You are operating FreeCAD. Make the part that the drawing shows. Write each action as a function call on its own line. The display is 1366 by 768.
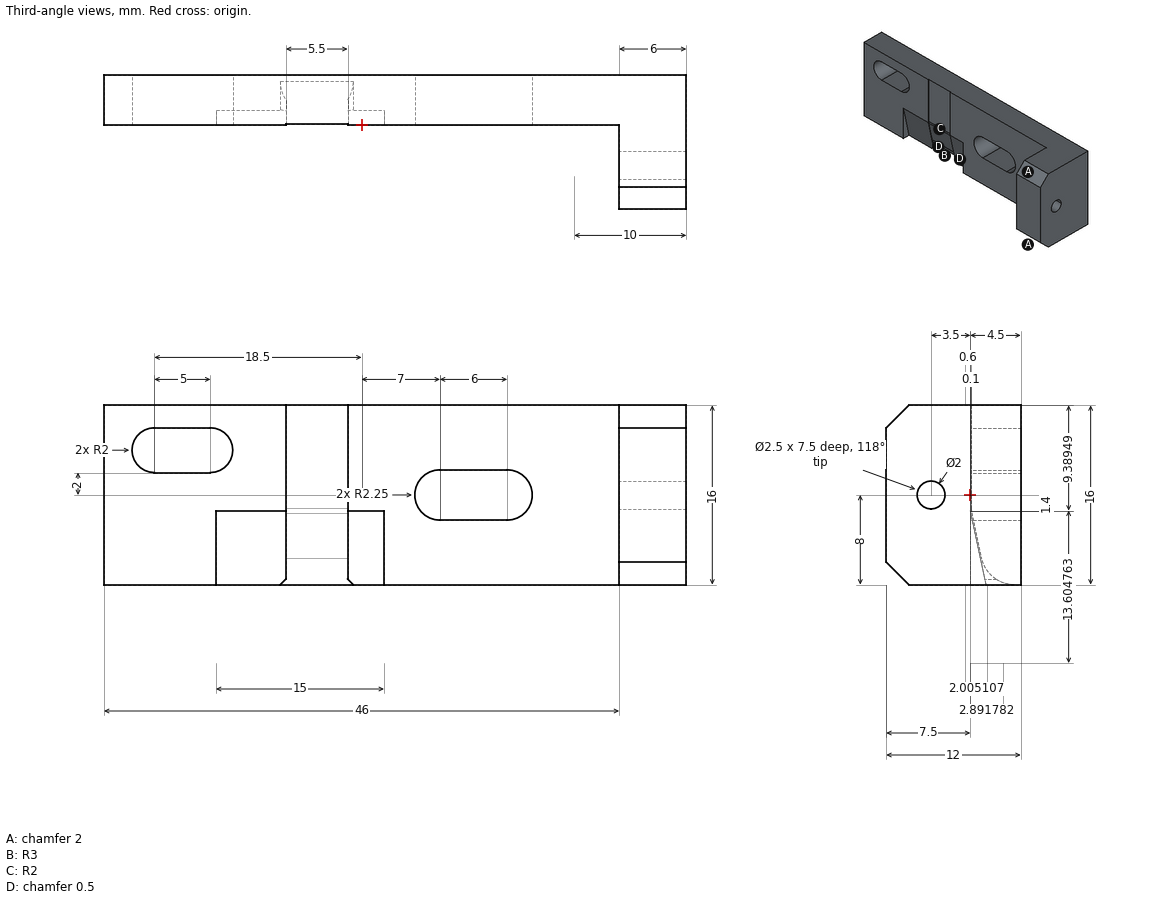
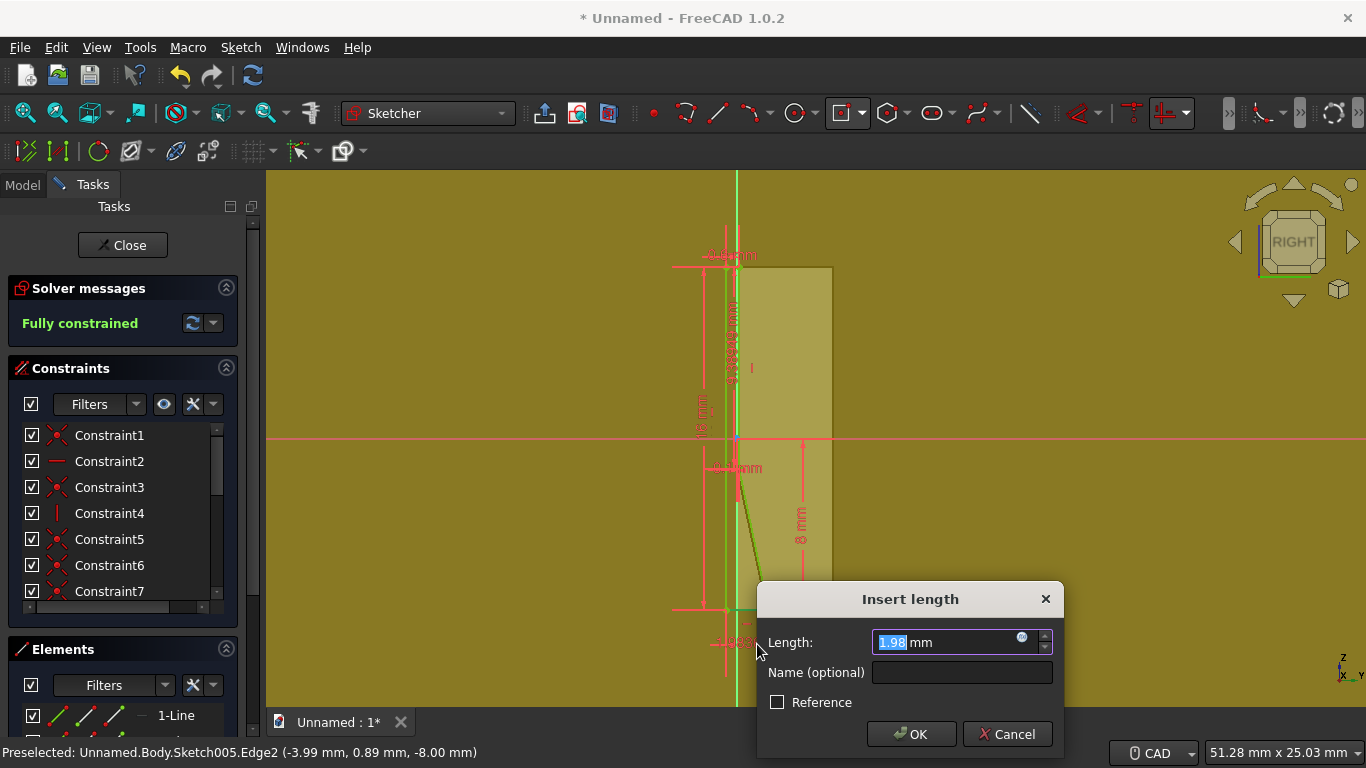
text(2.005107)
key(Return)
key(Escape)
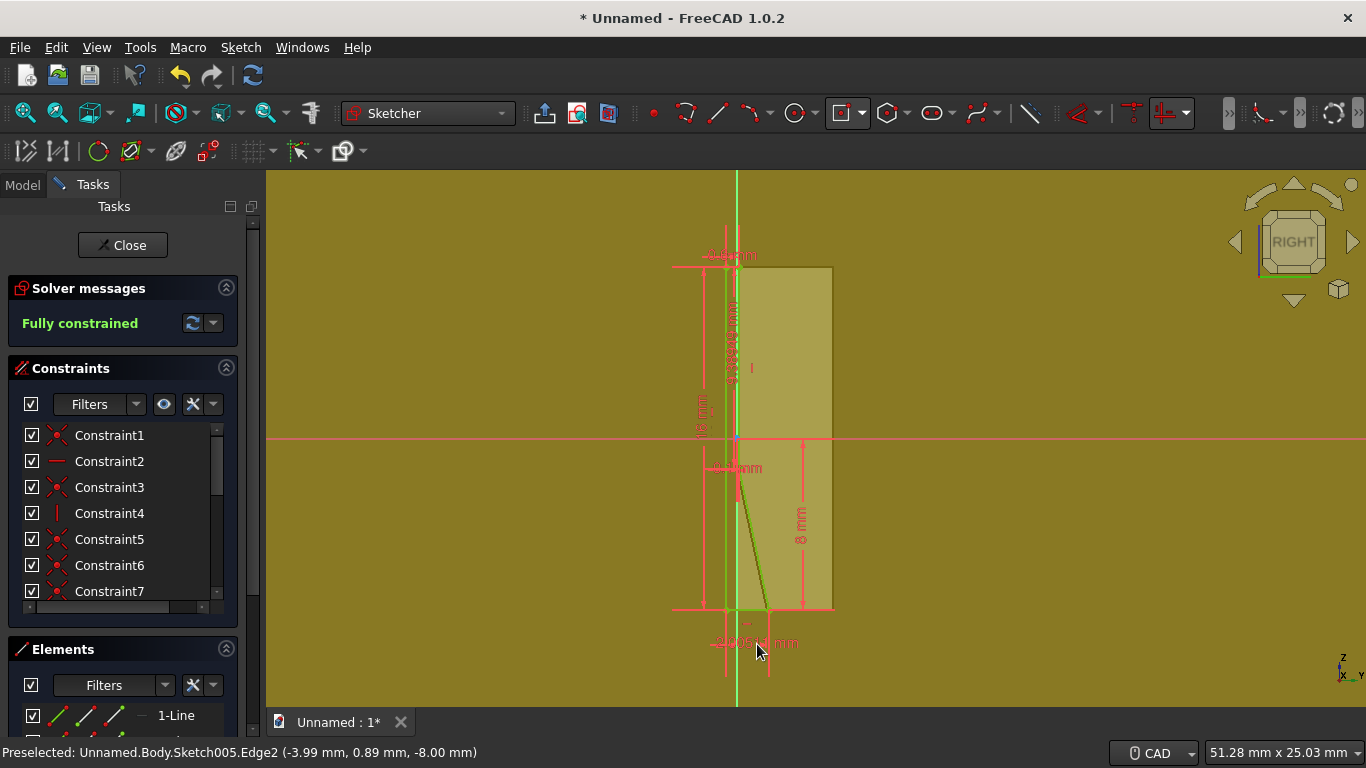
click(123, 245)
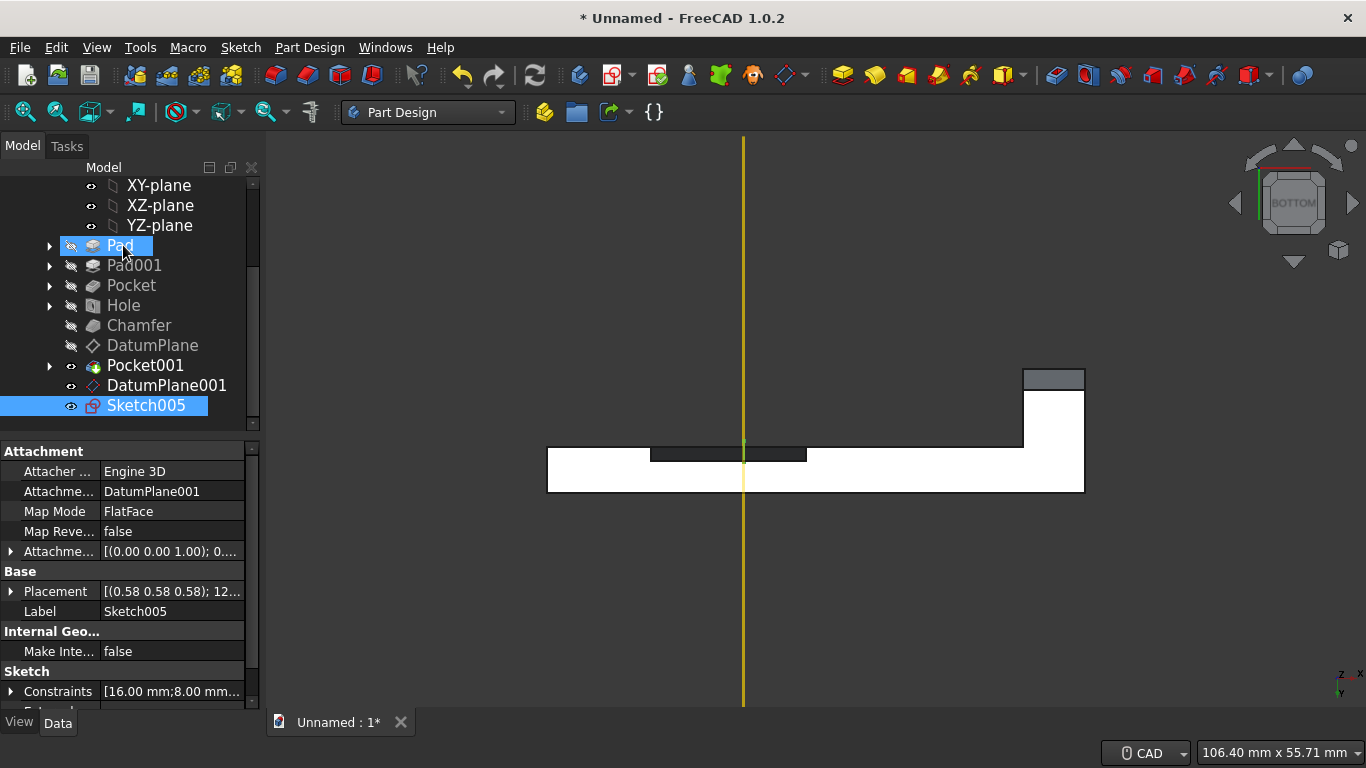
click(1058, 76)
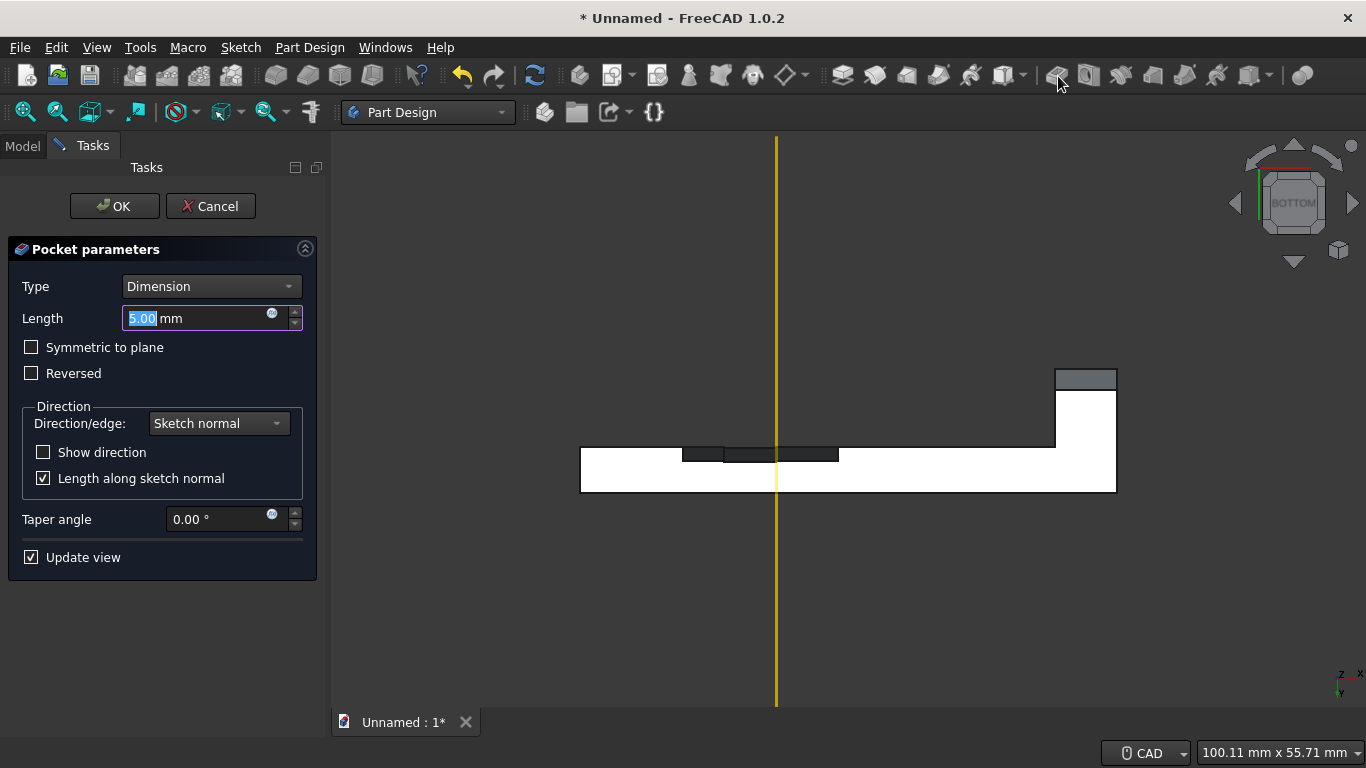
text(5.5)
key(Tab)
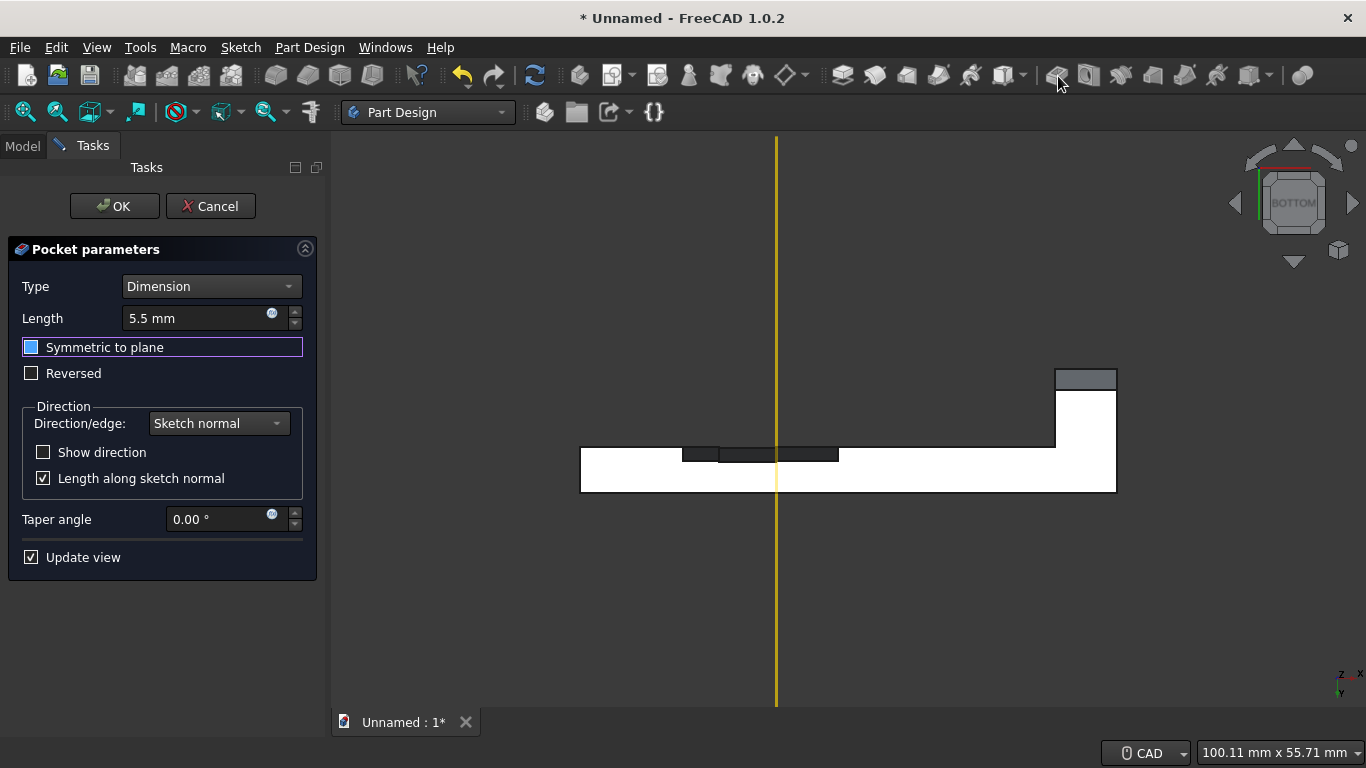
click(30, 347)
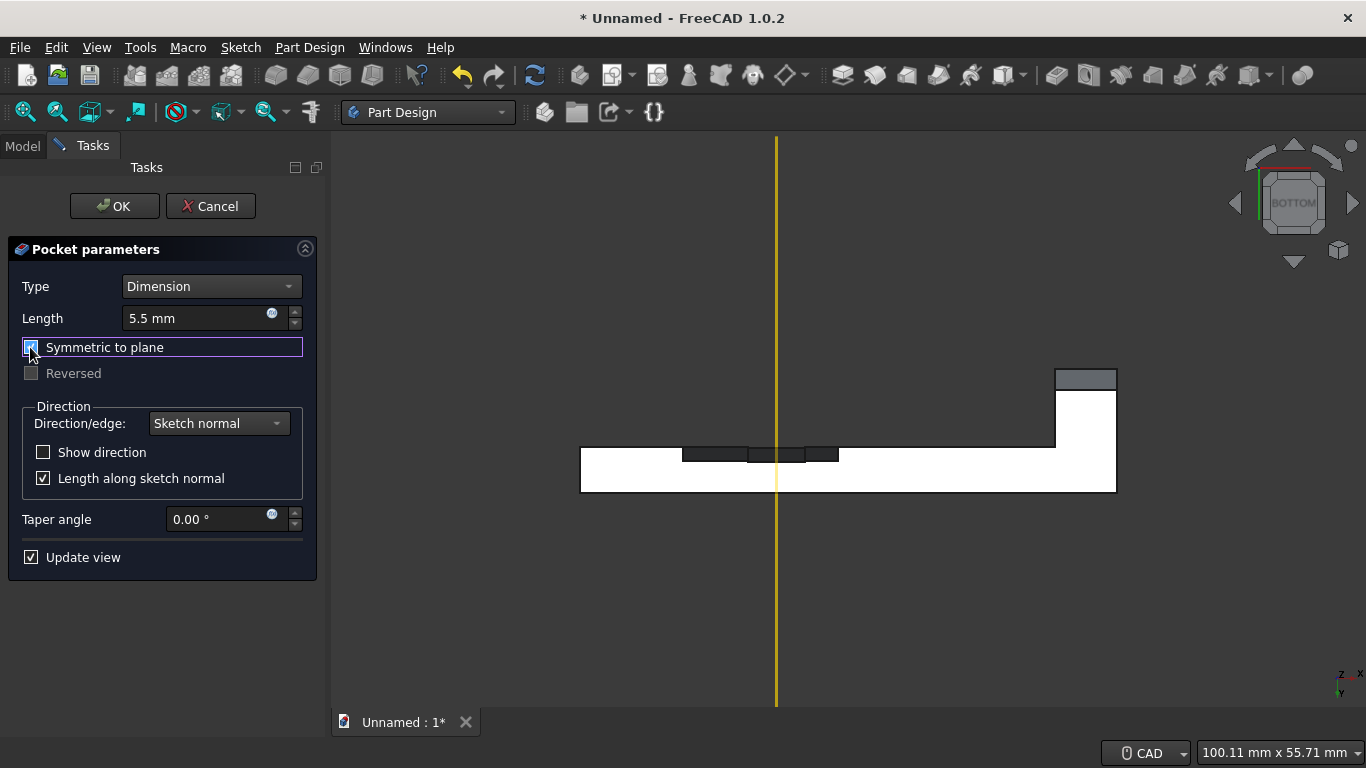
click(115, 206)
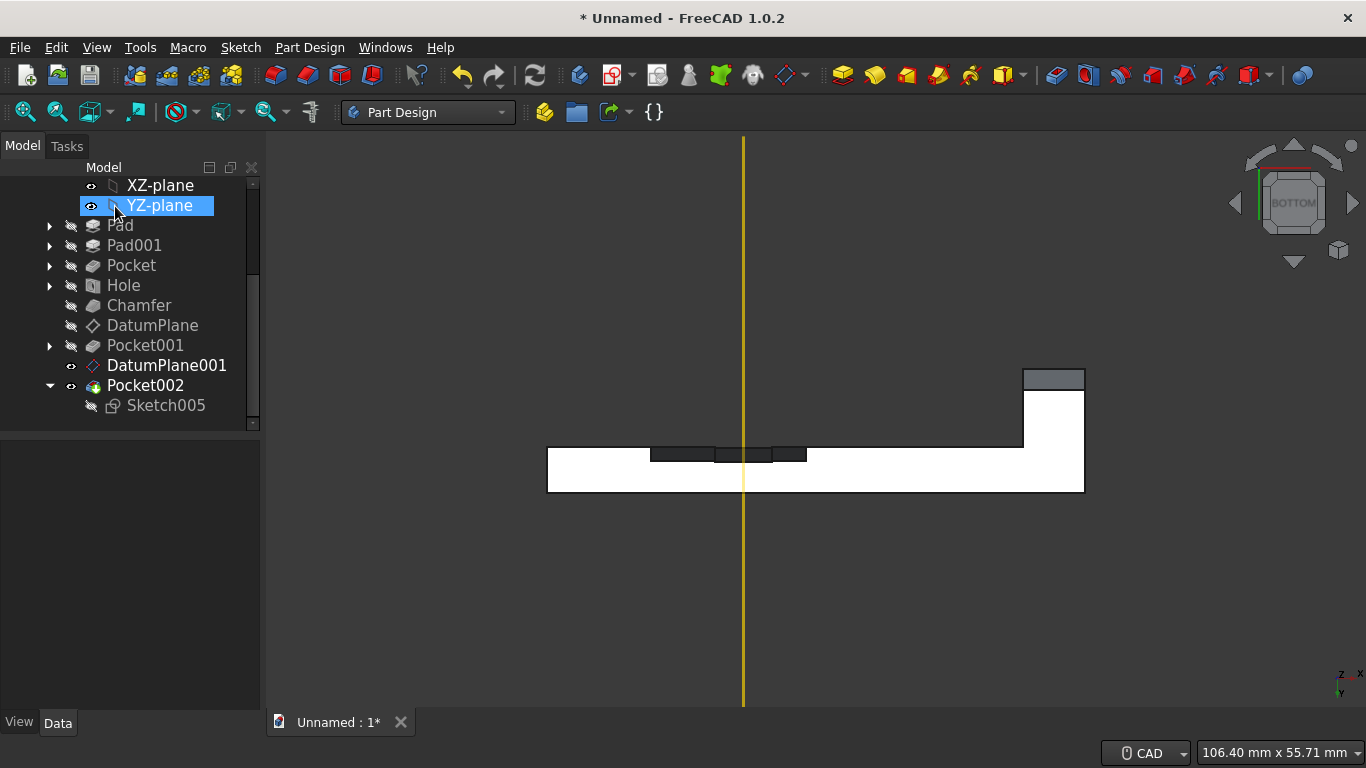
click(116, 366)
key(space)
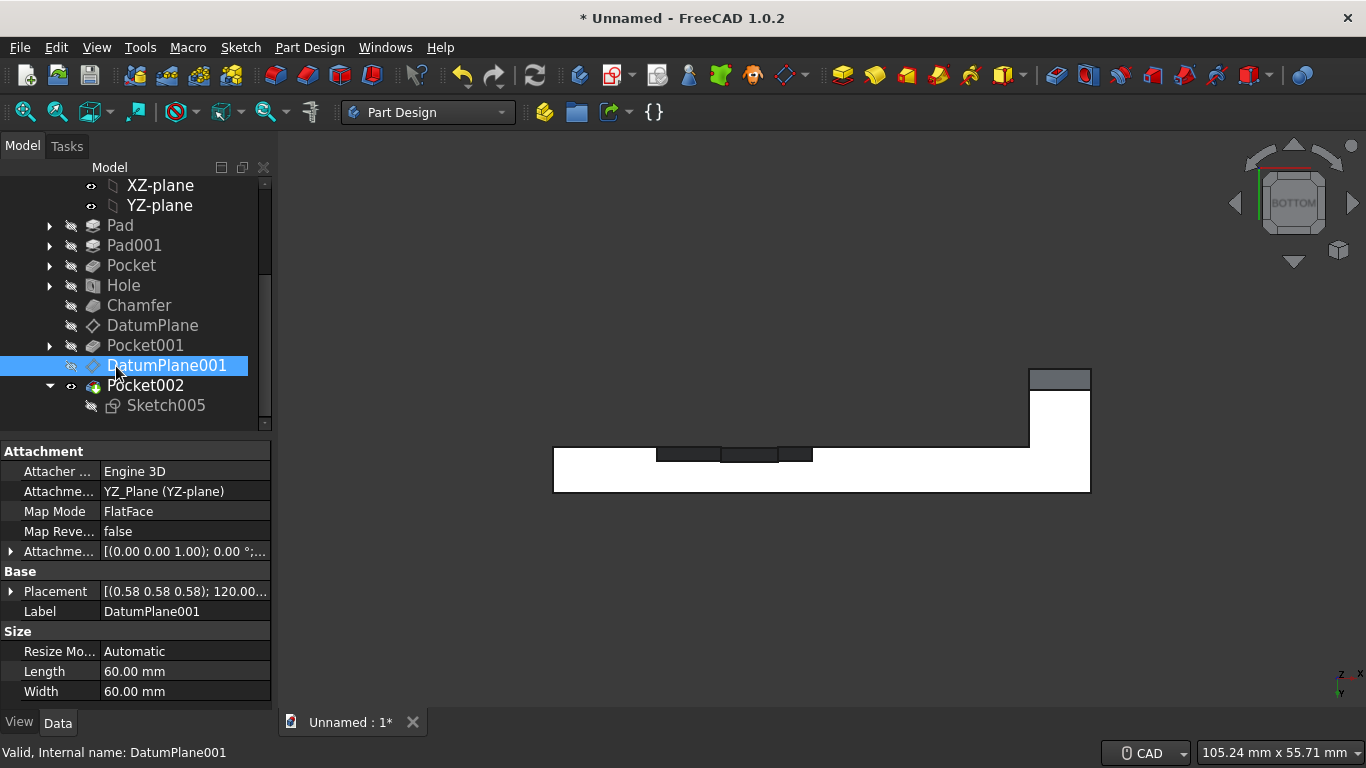
click(750, 461)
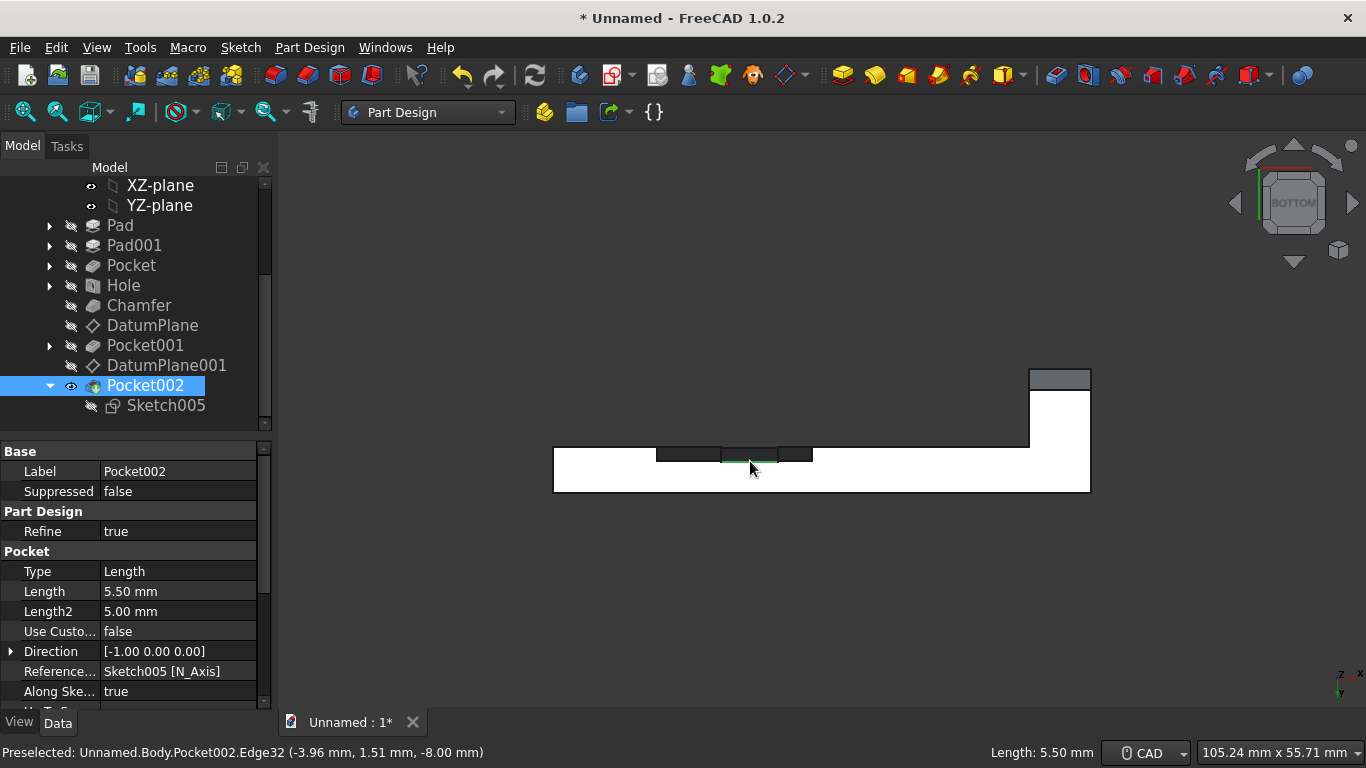
click(276, 76)